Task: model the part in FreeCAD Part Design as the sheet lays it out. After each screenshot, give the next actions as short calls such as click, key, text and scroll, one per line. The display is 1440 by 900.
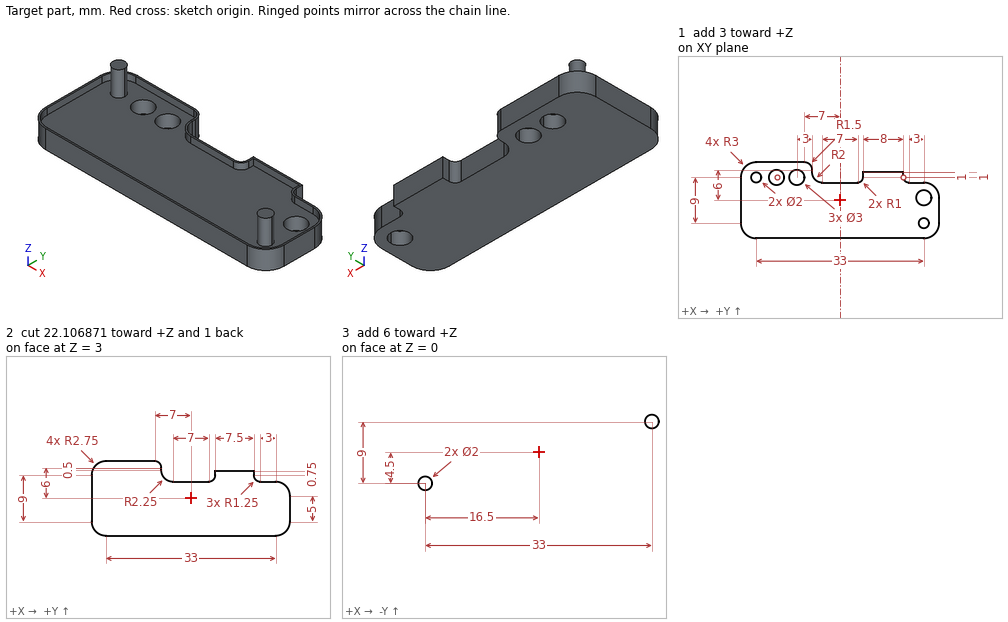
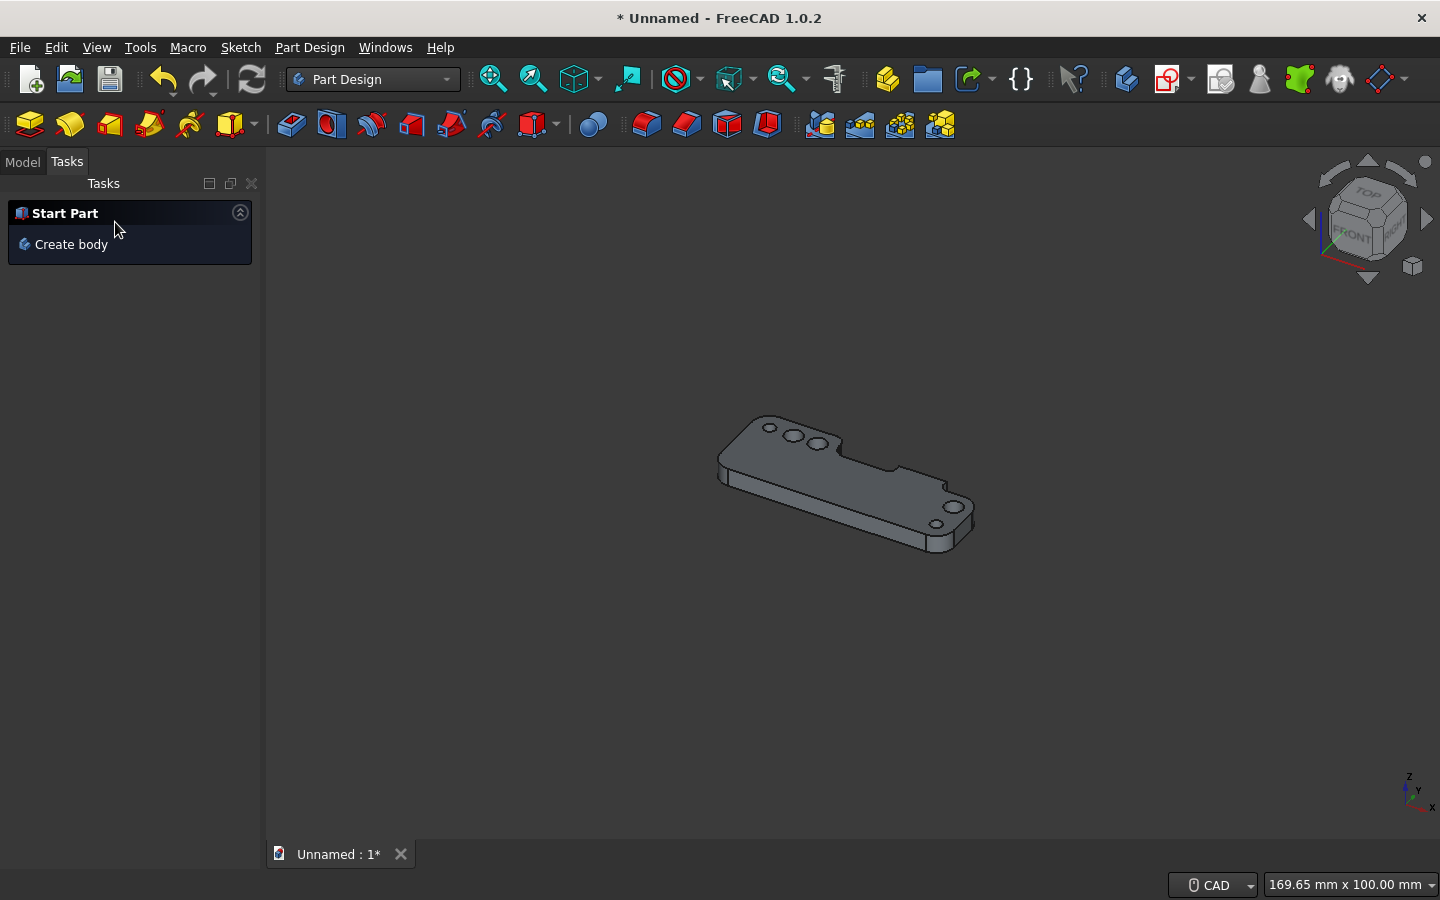
click(494, 80)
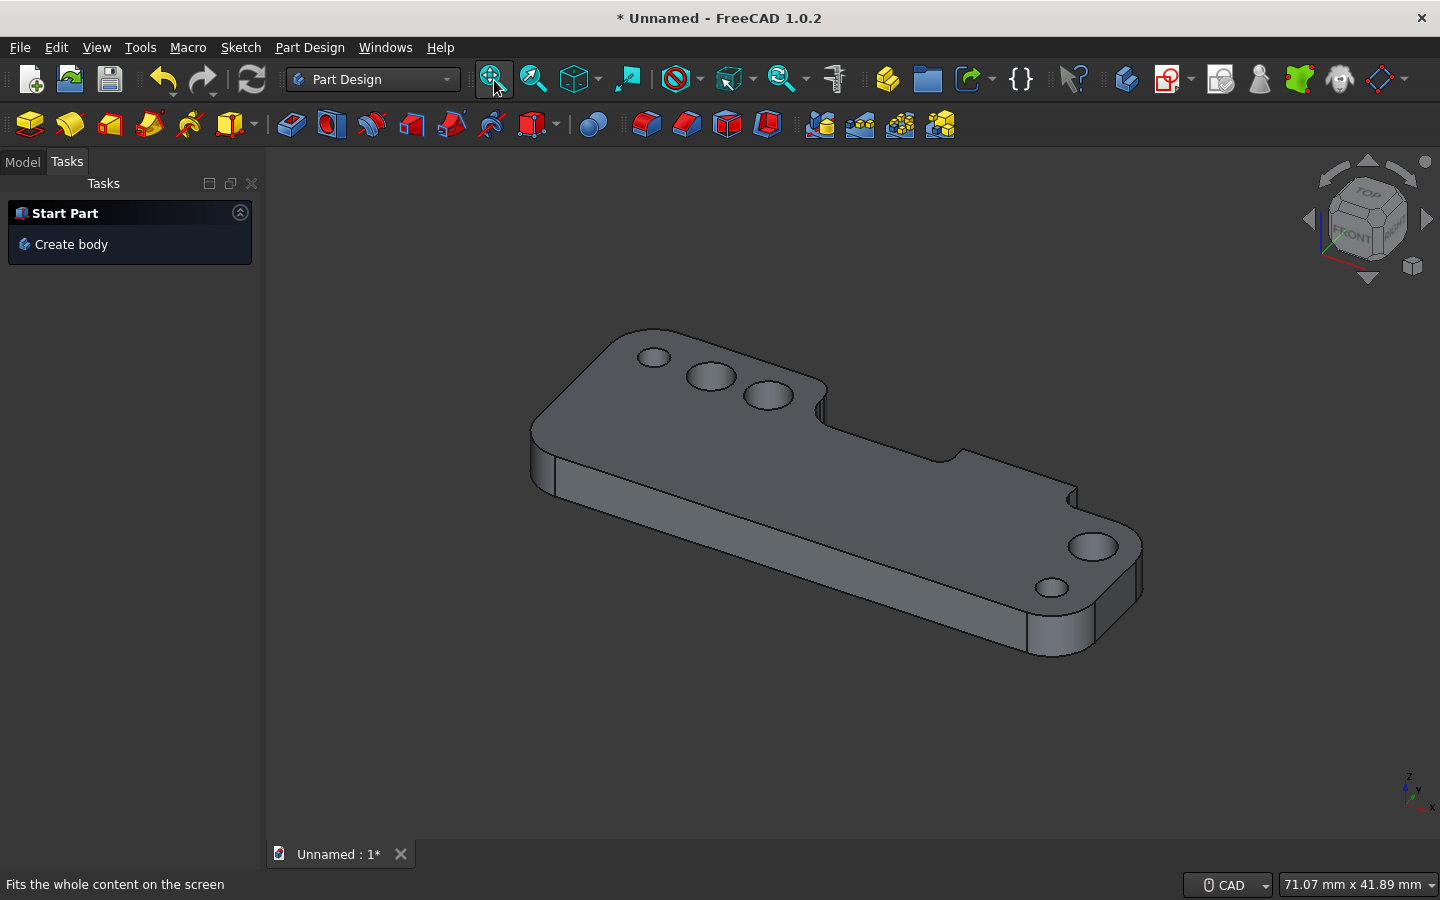
click(915, 516)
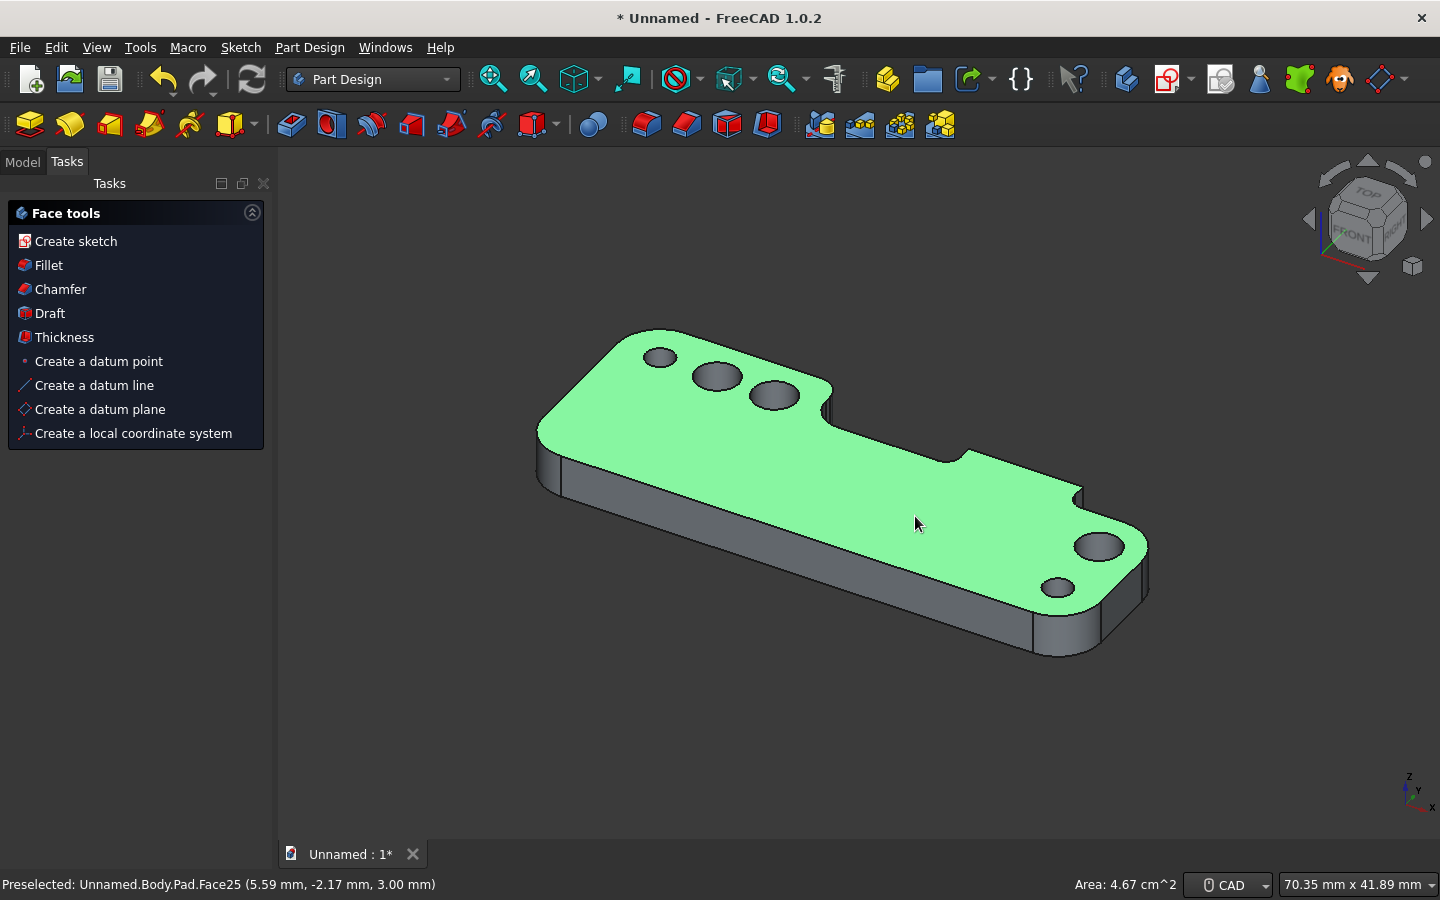
click(1168, 80)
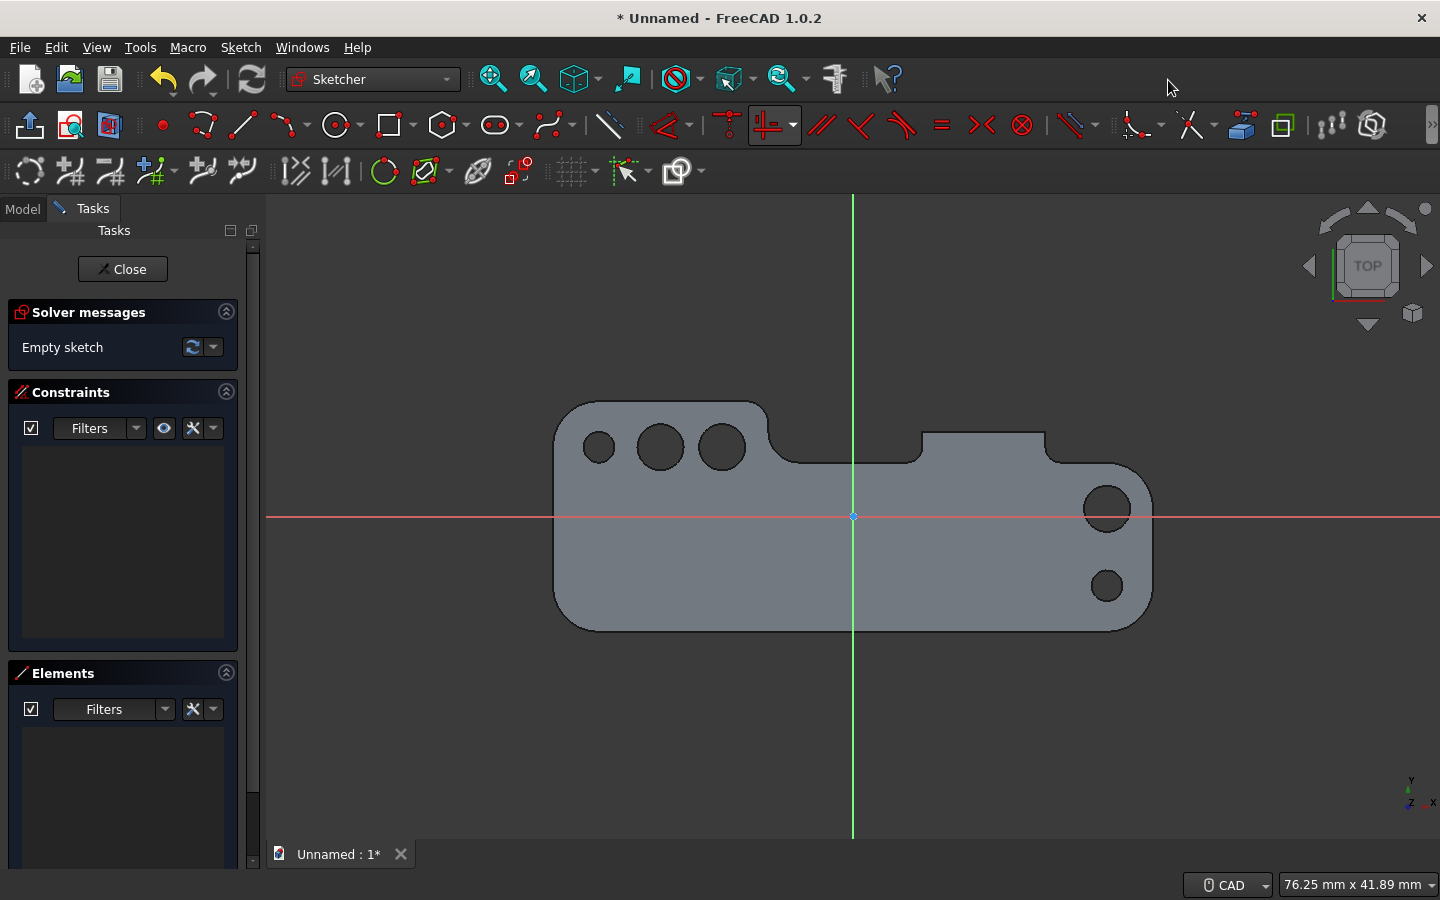
click(244, 126)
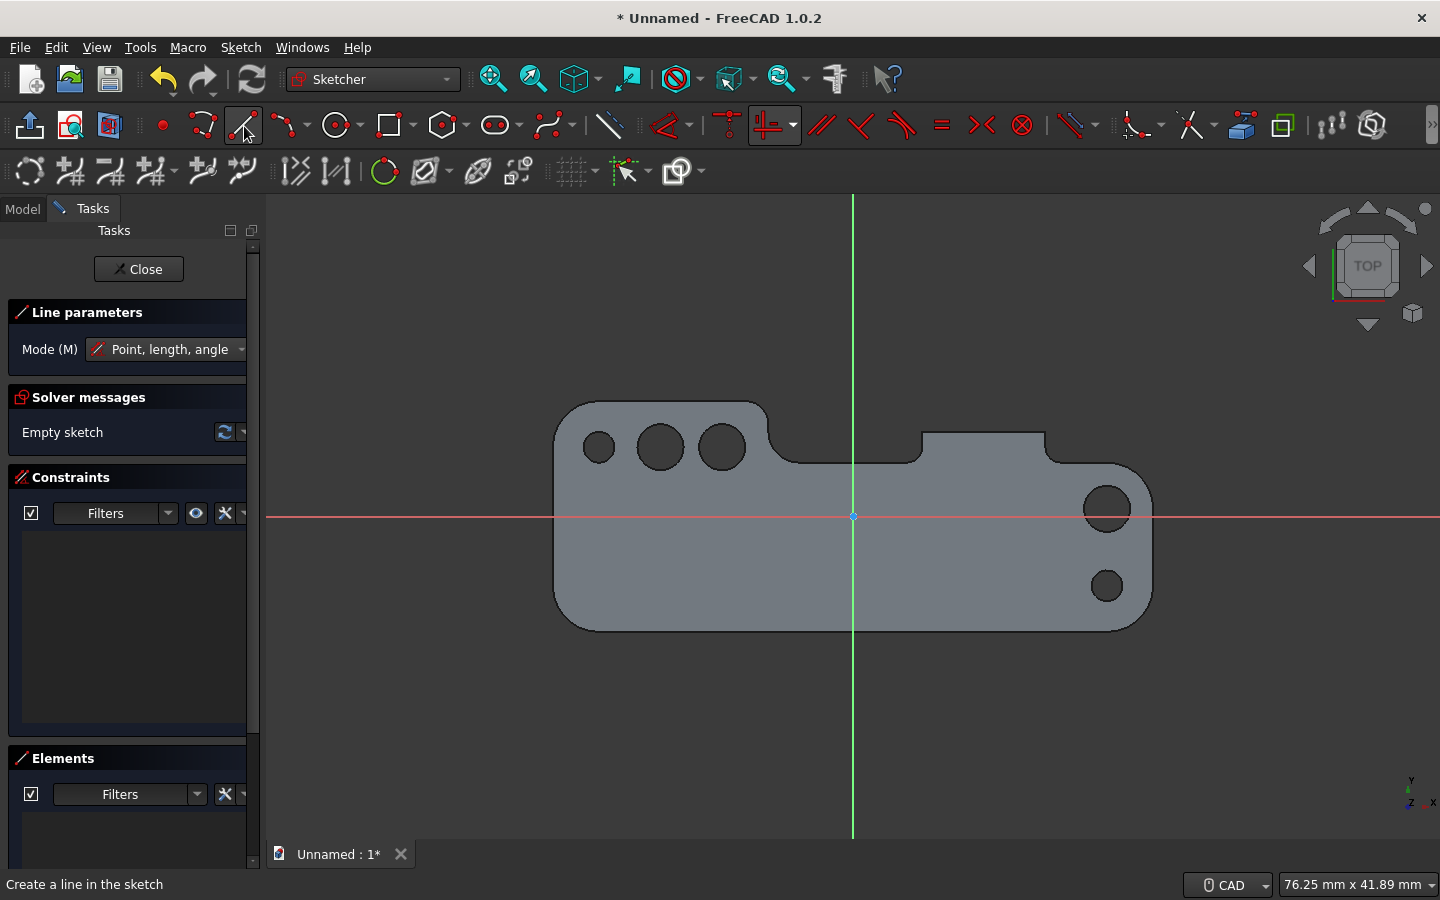
click(1107, 466)
click(1061, 466)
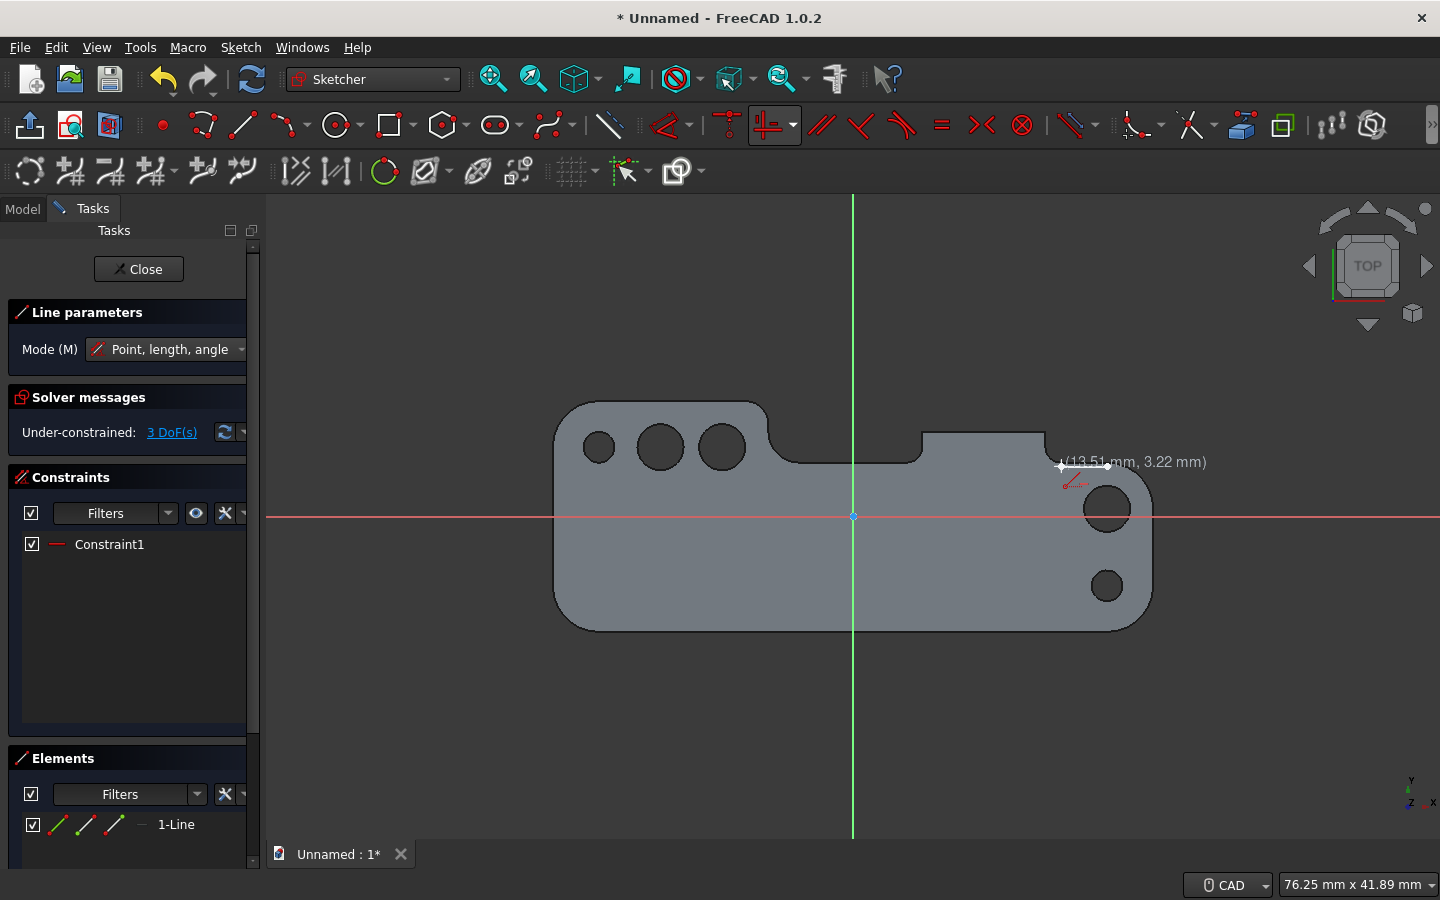
click(204, 126)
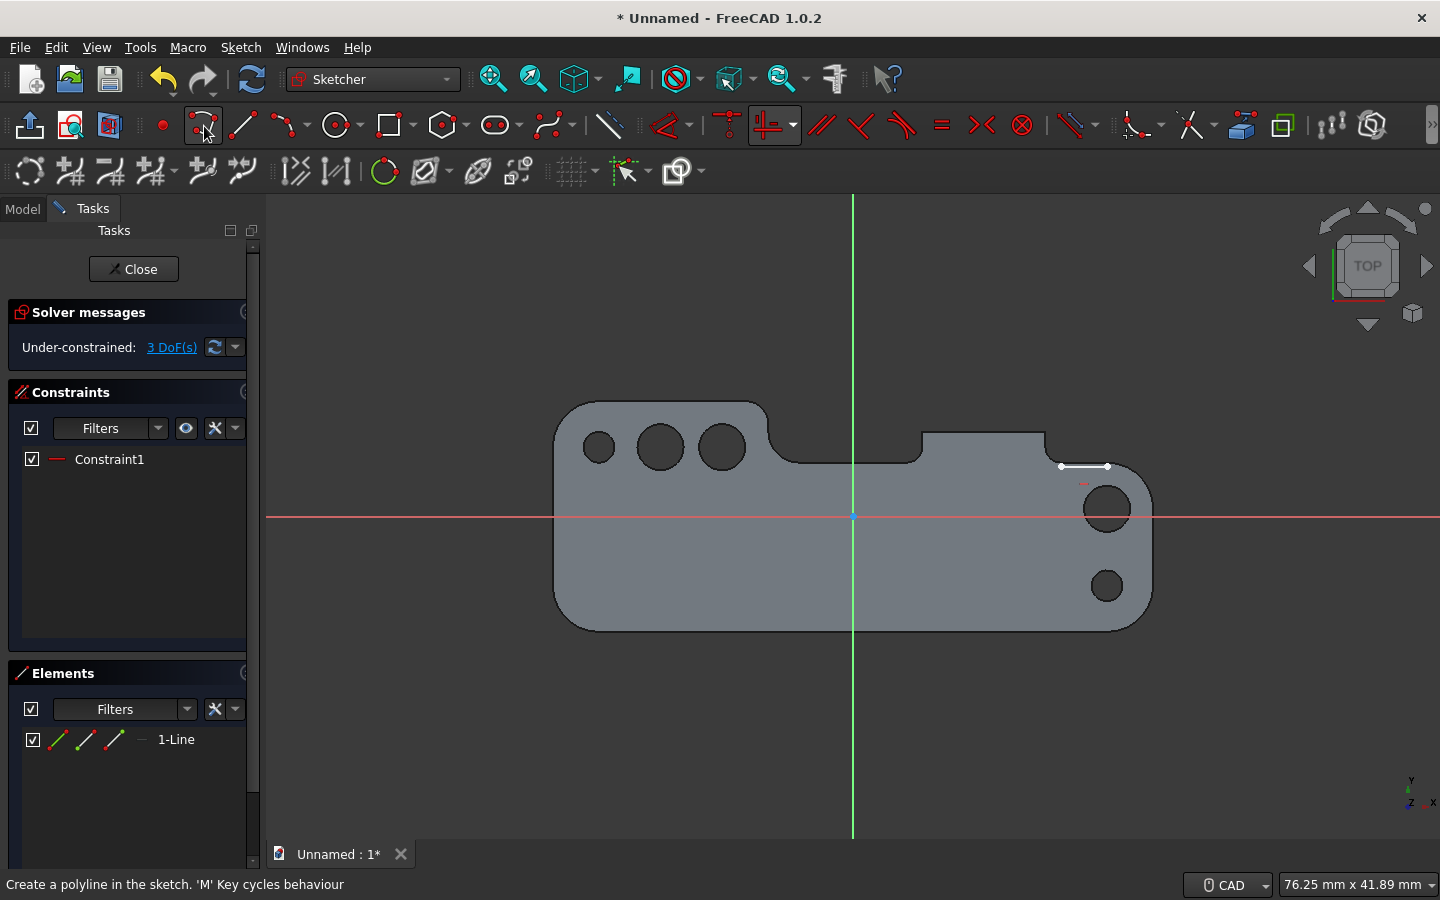
click(1042, 447)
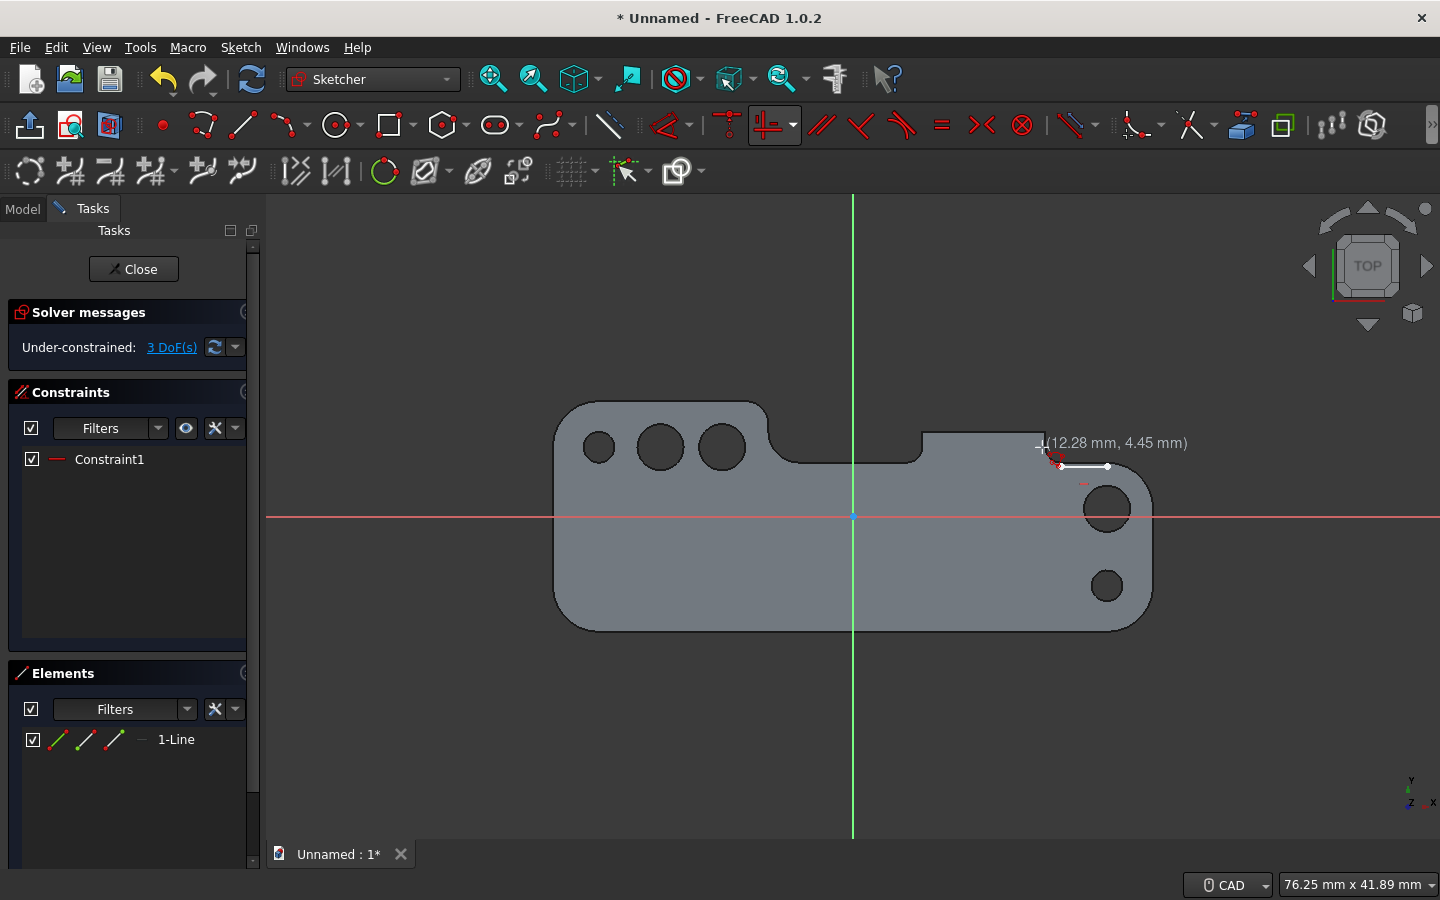
scroll(1042, 436, up, 2)